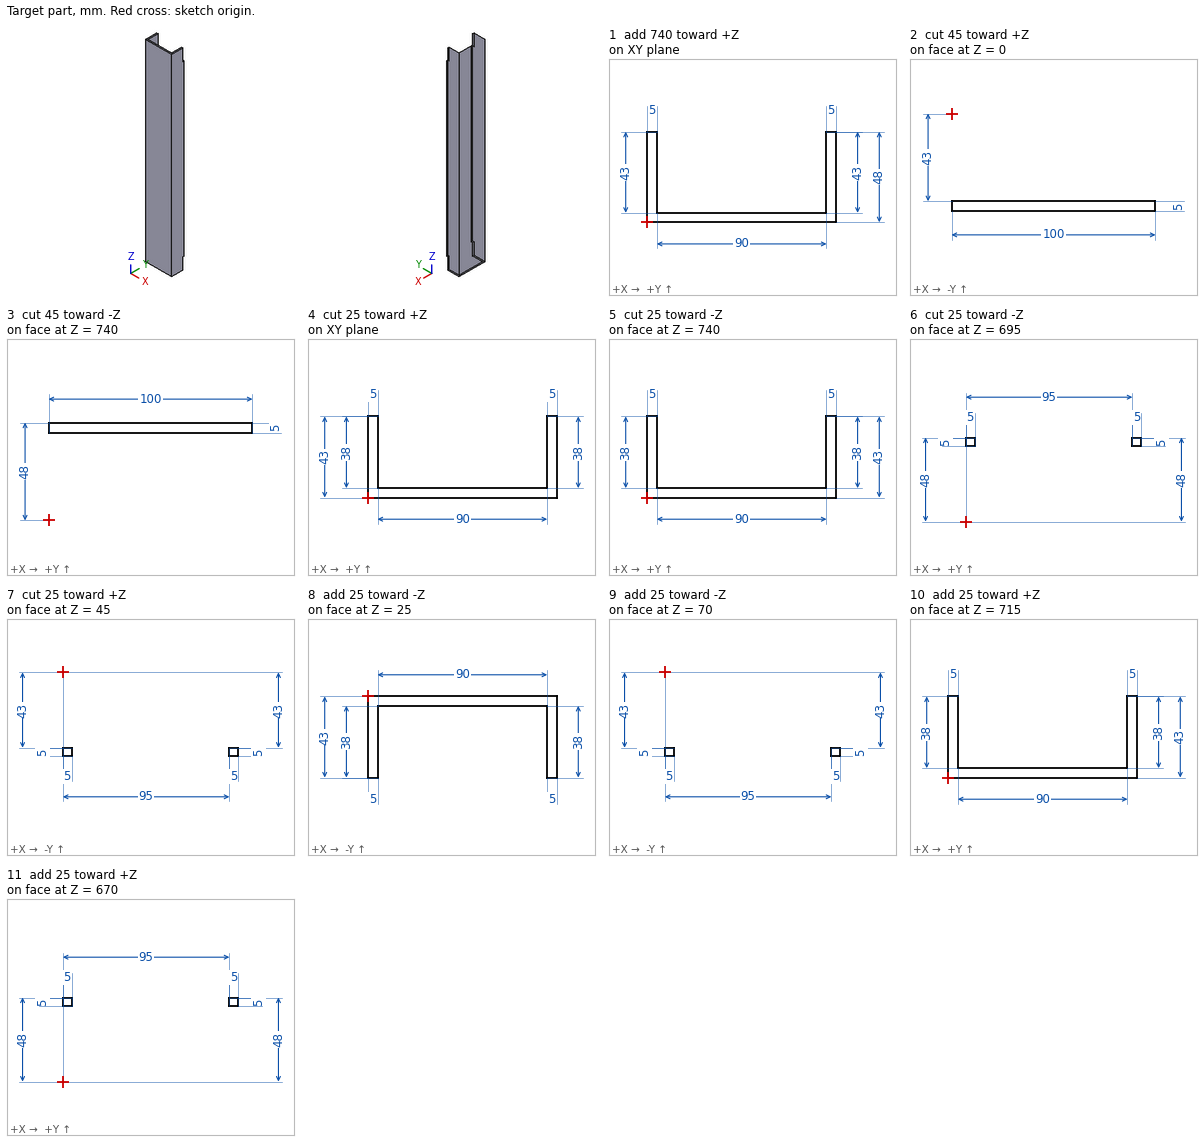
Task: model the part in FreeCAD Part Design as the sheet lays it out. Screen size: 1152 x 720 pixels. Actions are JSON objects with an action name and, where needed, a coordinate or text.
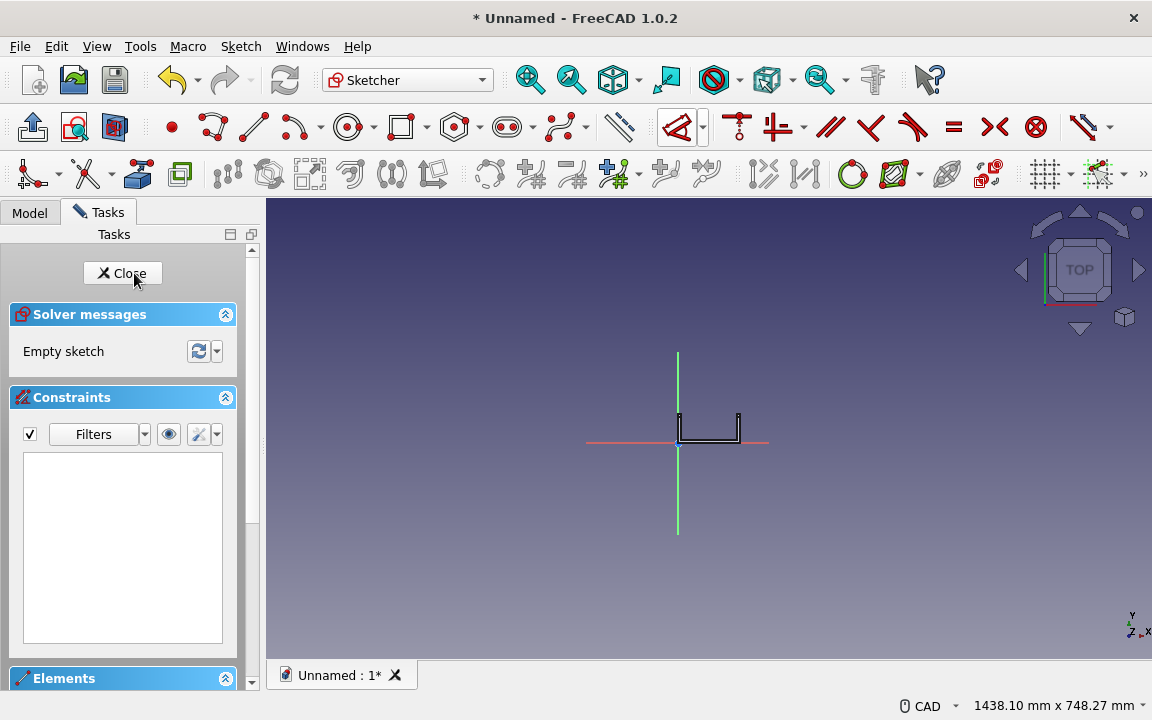
{"action": "left_click", "coordinate": [115, 128]}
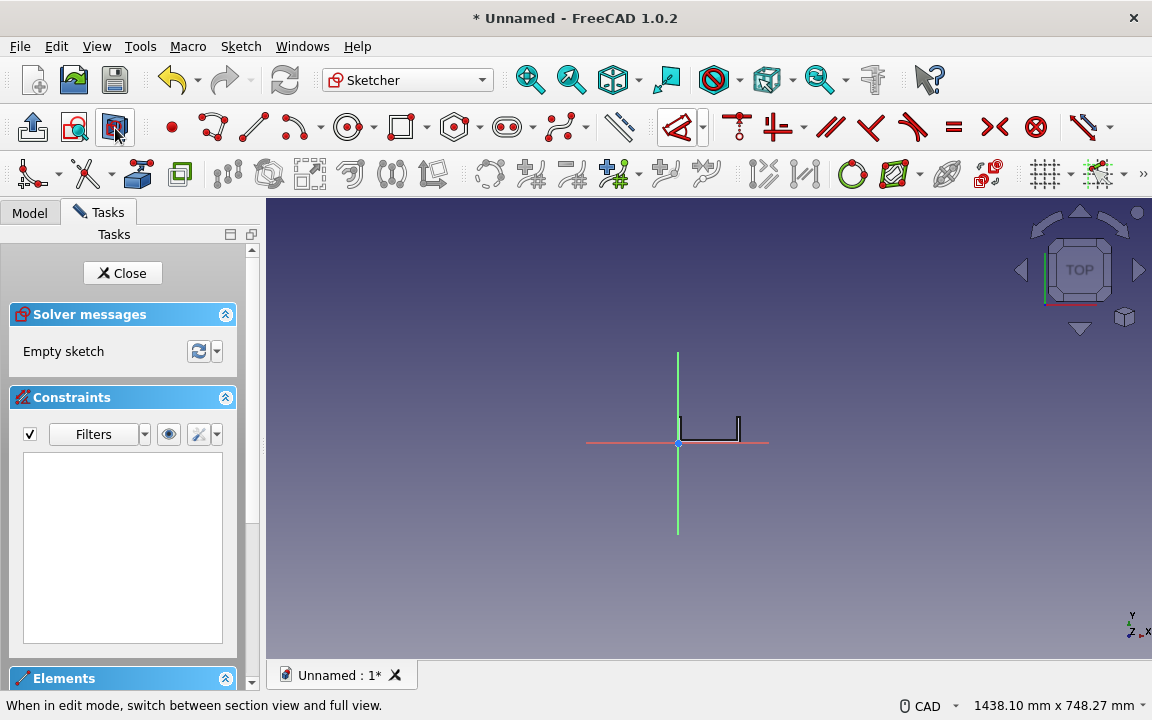
{"action": "scroll", "coordinate": [720, 430], "scroll_direction": "up", "scroll_amount": 10}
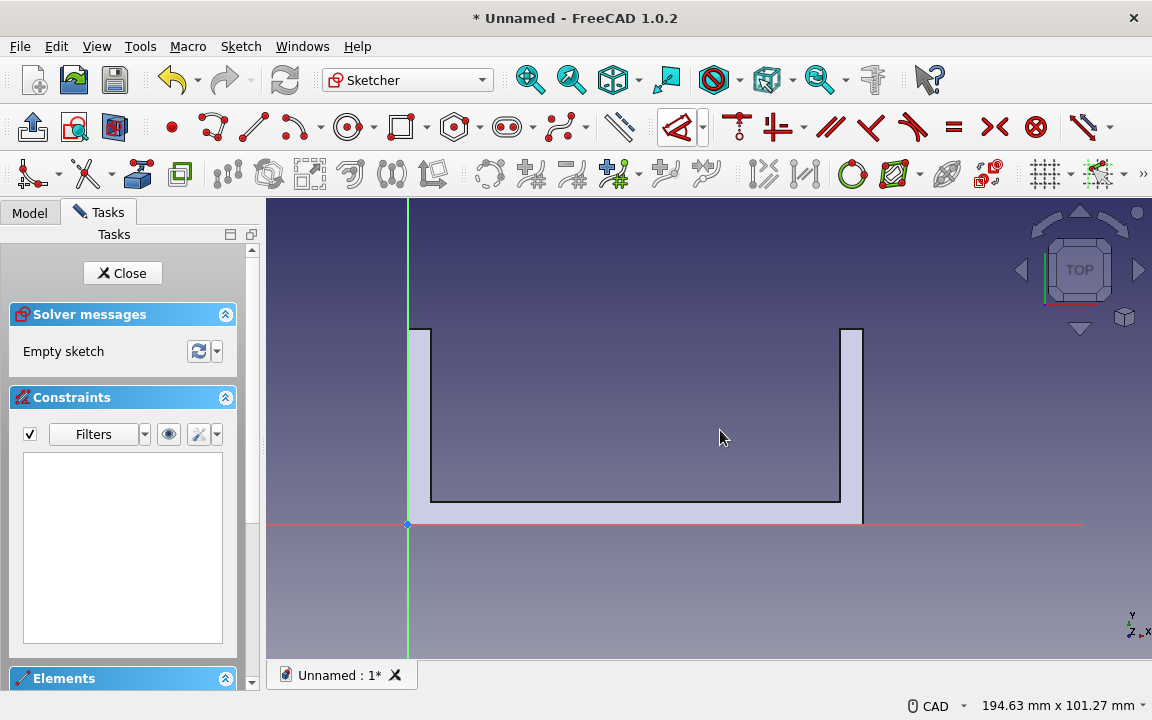
{"action": "left_click", "coordinate": [213, 128]}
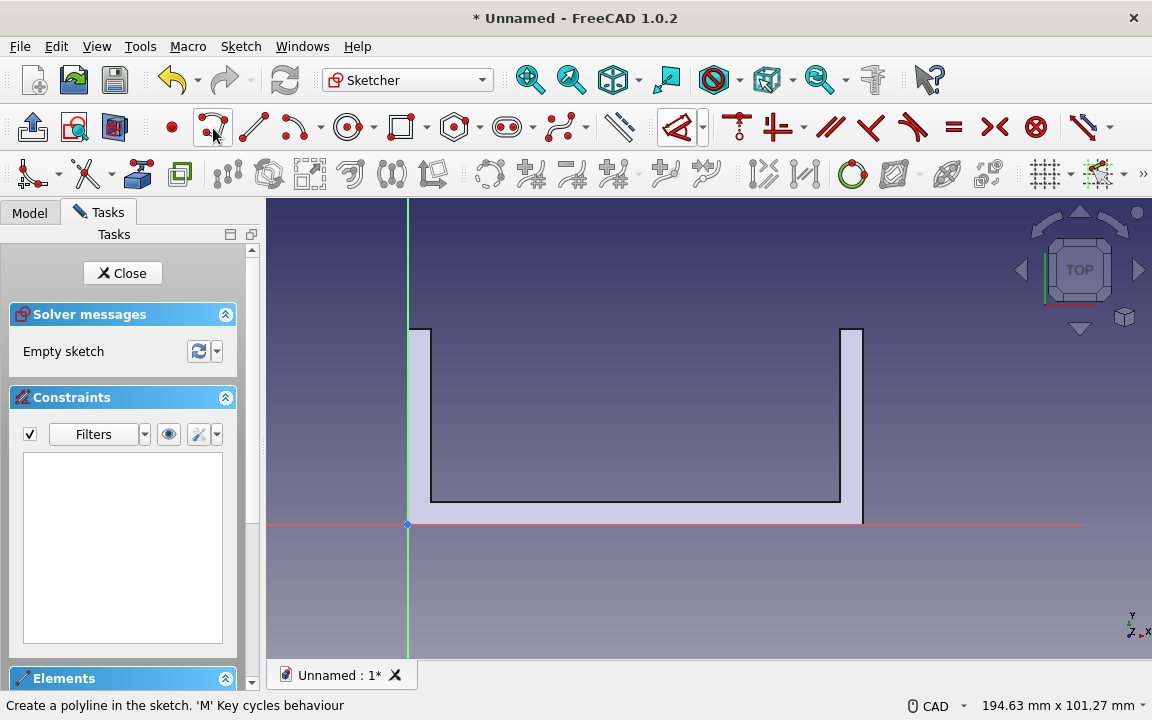
{"action": "left_click", "coordinate": [408, 525]}
{"action": "left_click", "coordinate": [417, 329]}
{"action": "left_click", "coordinate": [431, 329]}
{"action": "left_click", "coordinate": [431, 502]}
{"action": "left_click", "coordinate": [840, 502]}
{"action": "left_click", "coordinate": [840, 329]}
{"action": "left_click", "coordinate": [863, 329]}
{"action": "left_click", "coordinate": [863, 516]}
{"action": "left_click", "coordinate": [408, 525]}
{"action": "key", "text": "Escape"}
{"action": "key", "text": "Escape"}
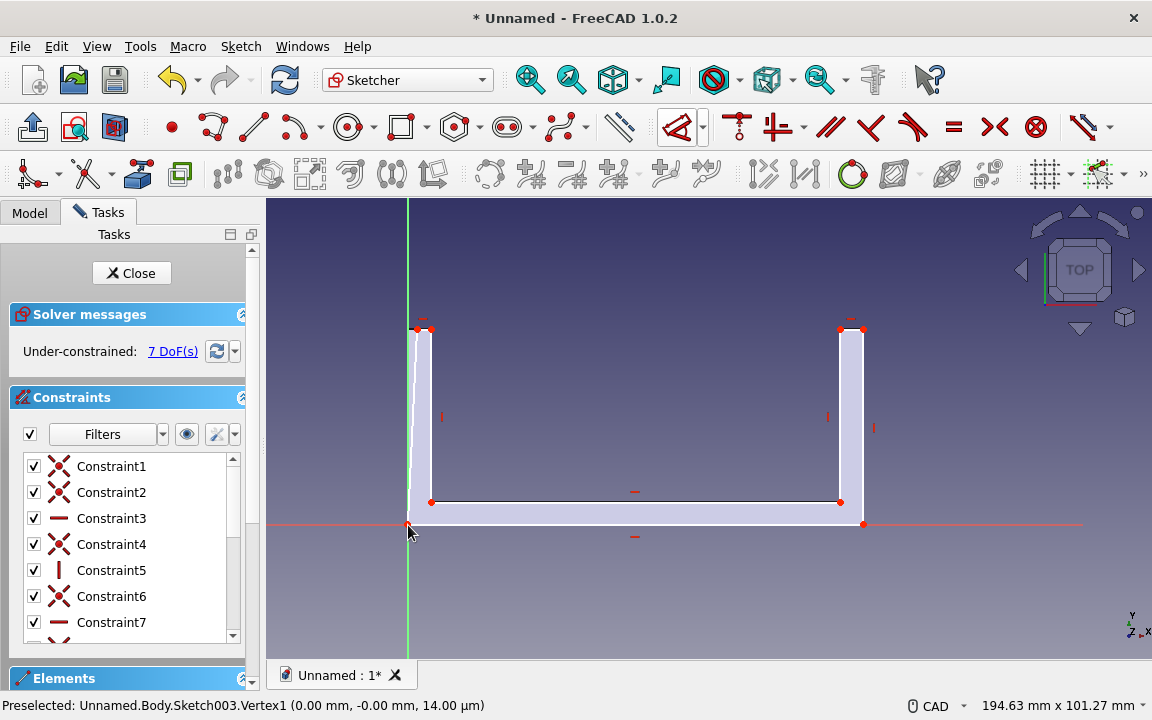
{"action": "left_click", "coordinate": [411, 466]}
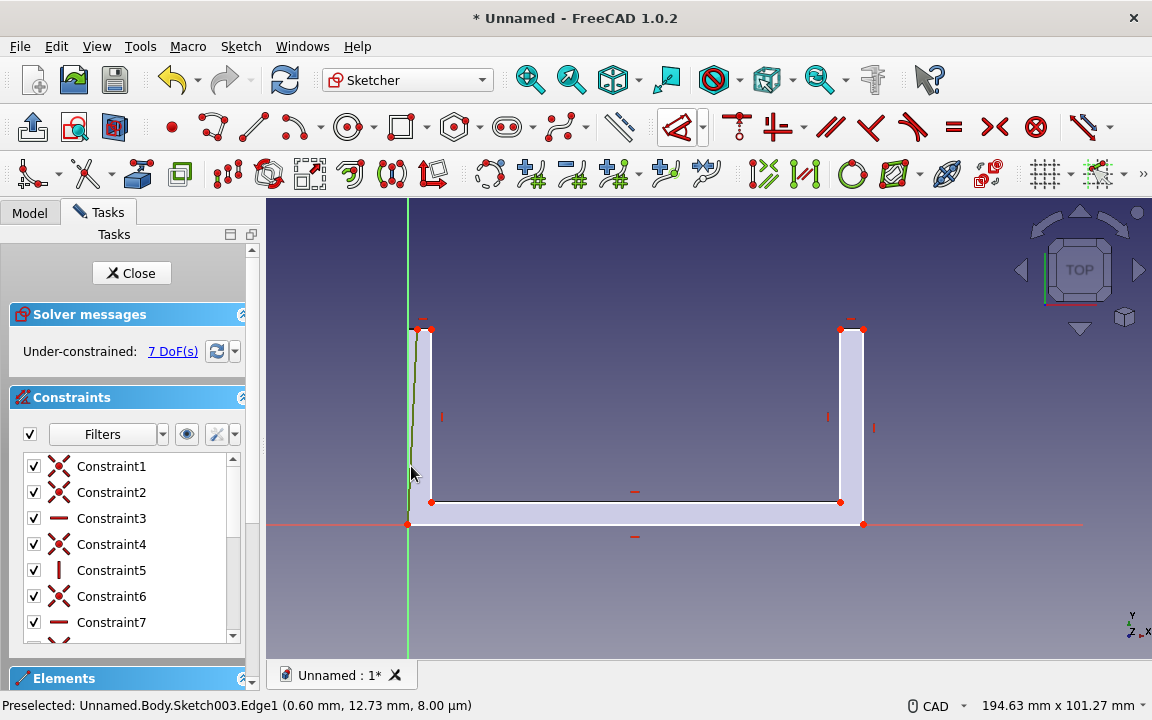
{"action": "left_click", "coordinate": [804, 128]}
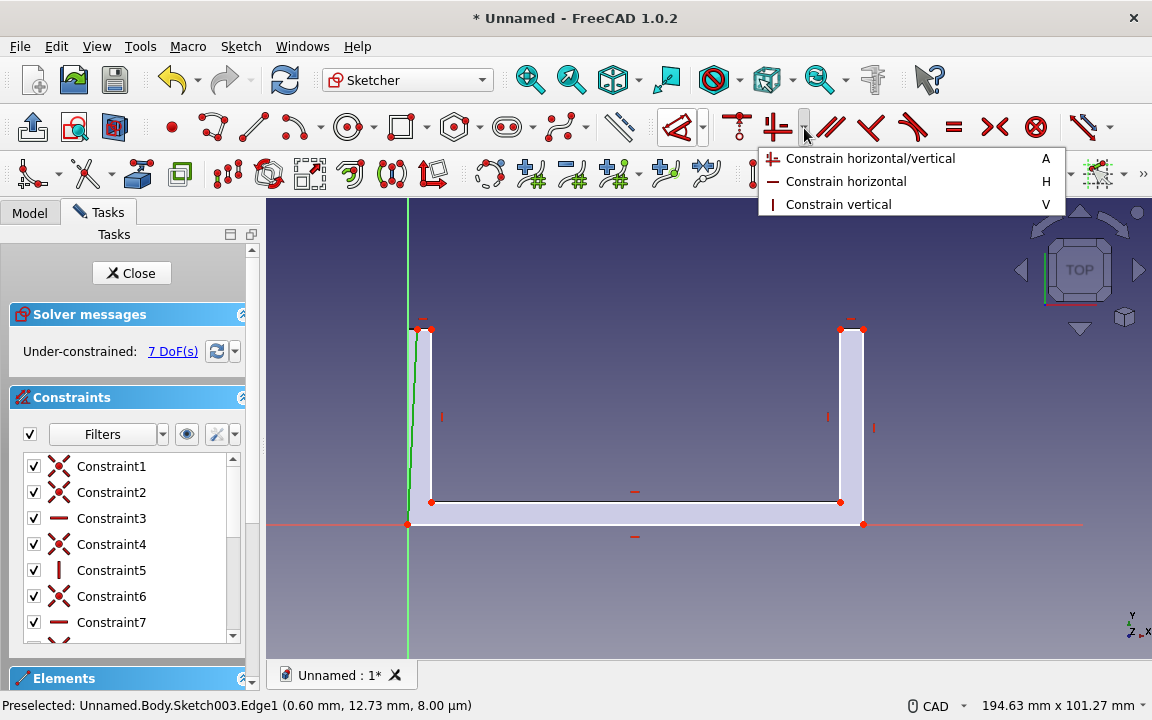
{"action": "left_click", "coordinate": [912, 204]}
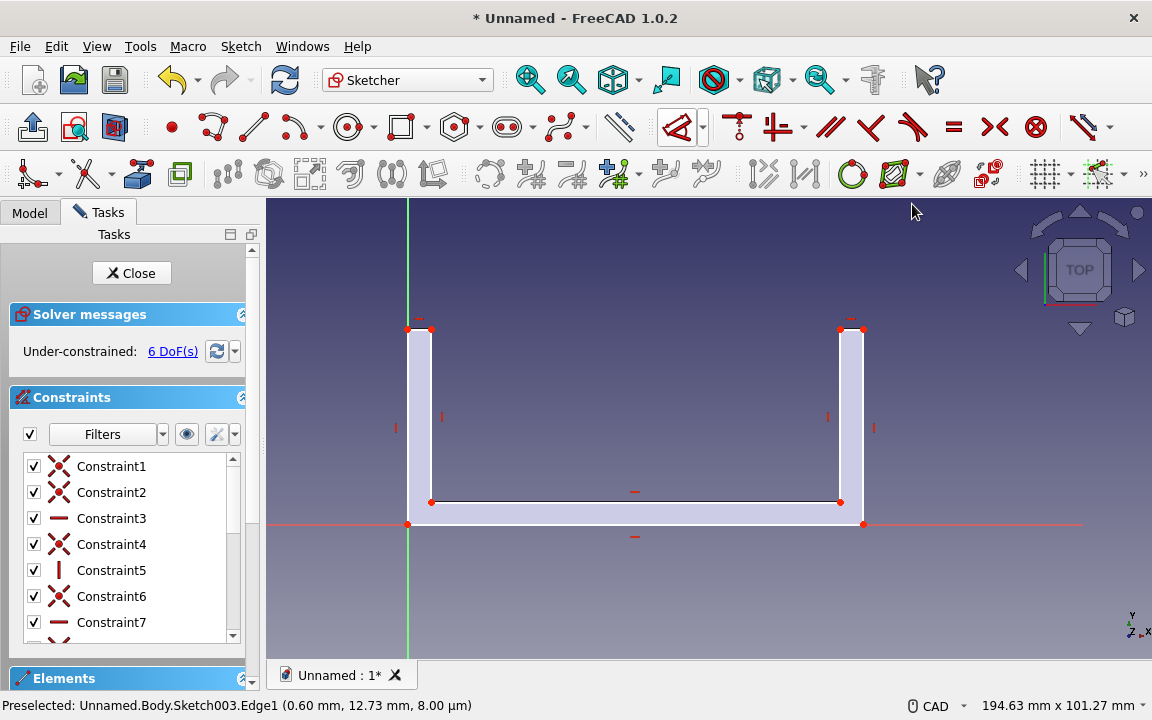
{"action": "scroll", "coordinate": [417, 330], "scroll_direction": "up", "scroll_amount": 3}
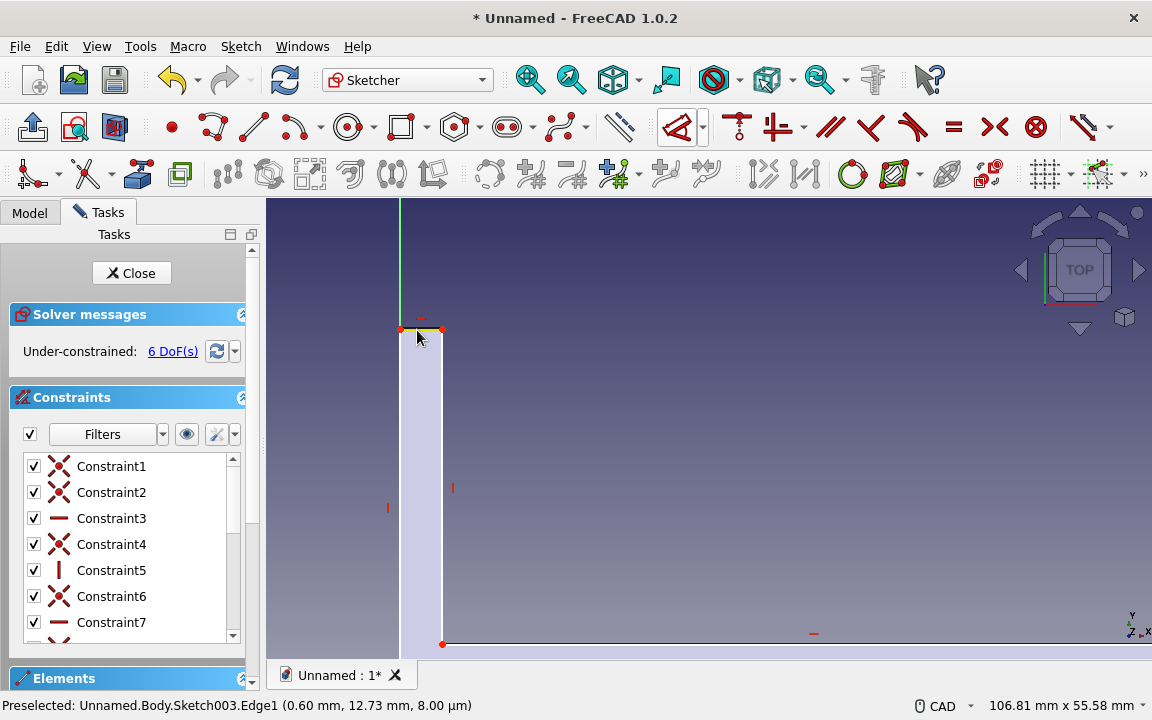
{"action": "left_click", "coordinate": [417, 330]}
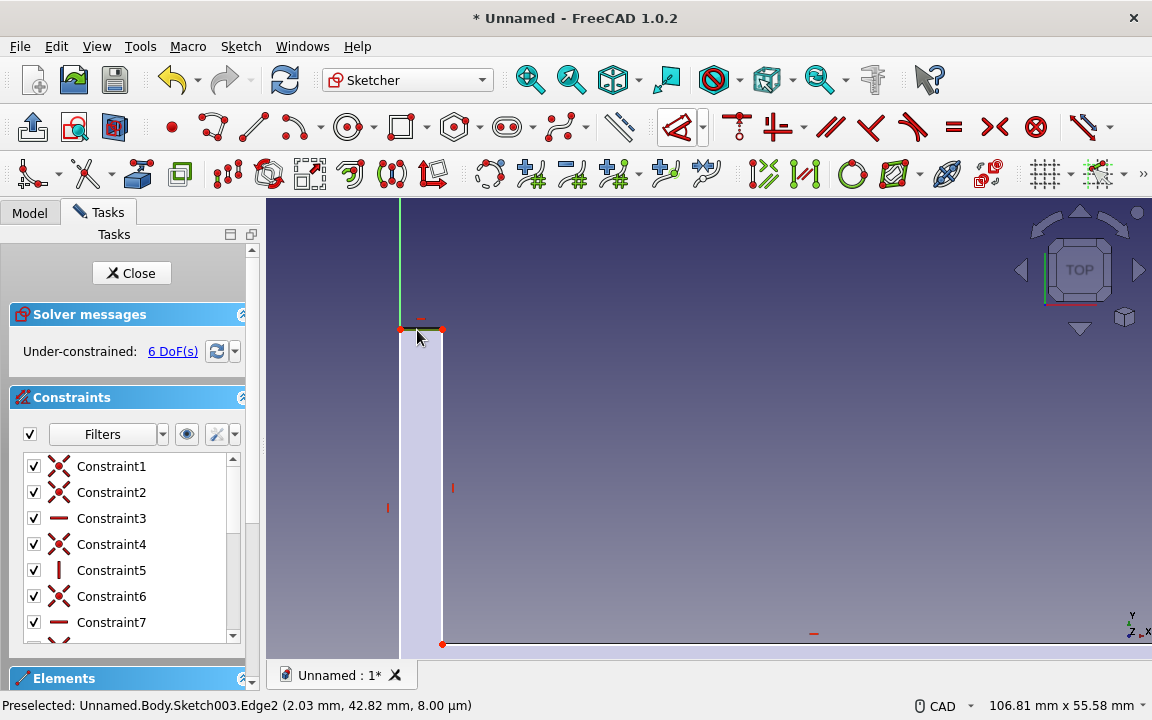
{"action": "key", "text": "l"}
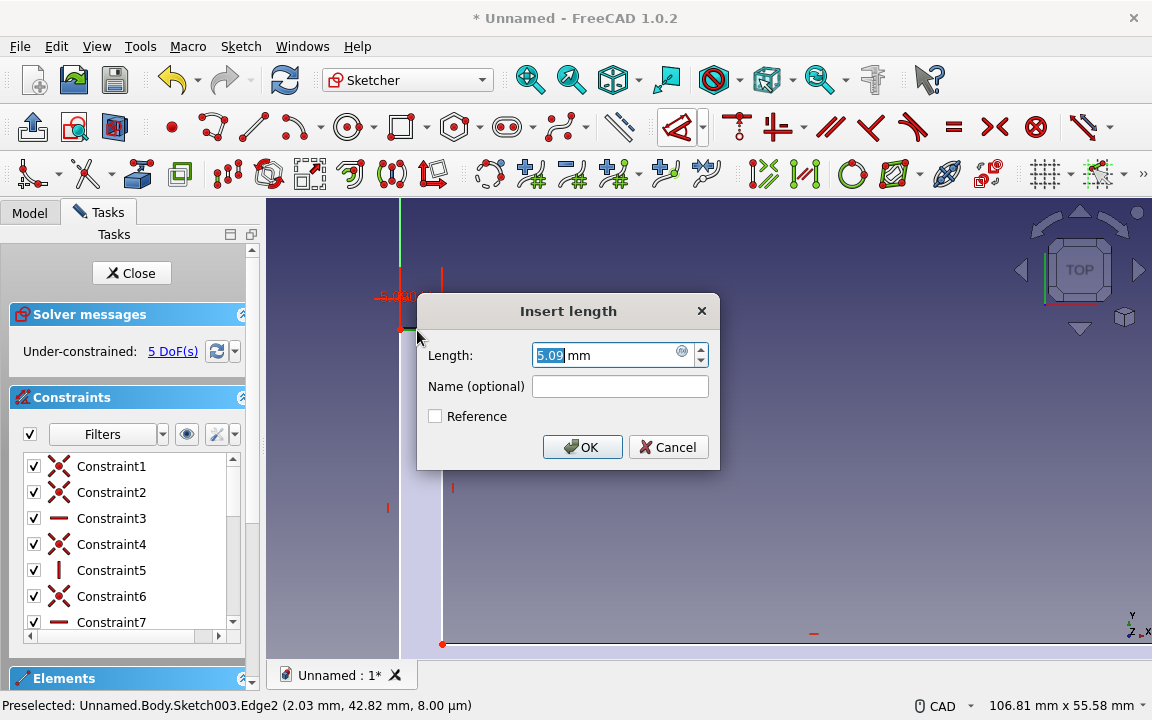
{"action": "type", "text": "5"}
{"action": "key", "text": "Return"}